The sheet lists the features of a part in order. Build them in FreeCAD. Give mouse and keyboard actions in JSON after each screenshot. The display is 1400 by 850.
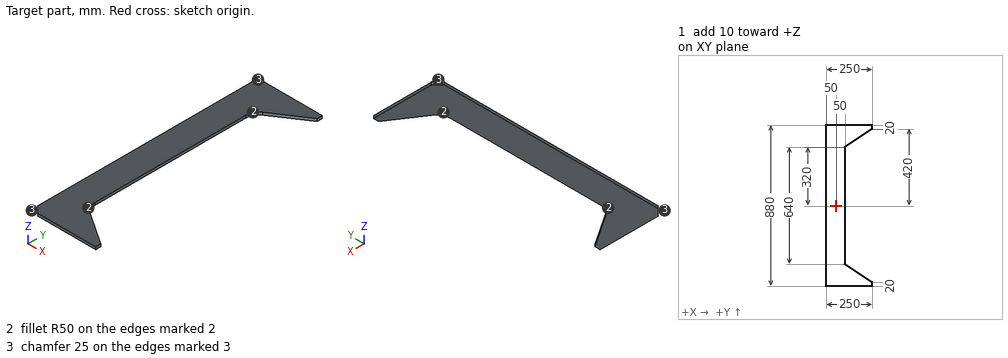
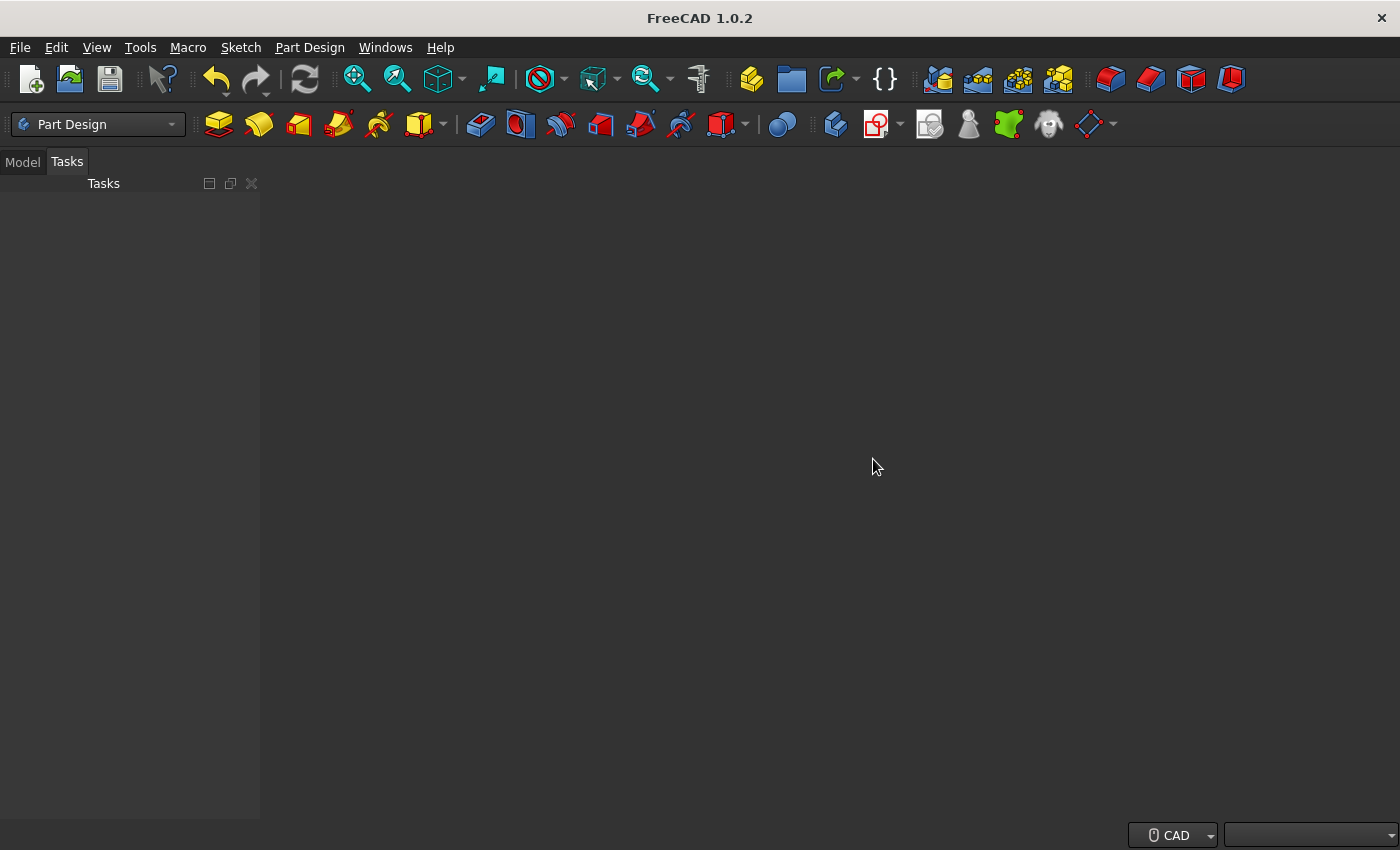
{"action": "key", "text": "ctrl+n"}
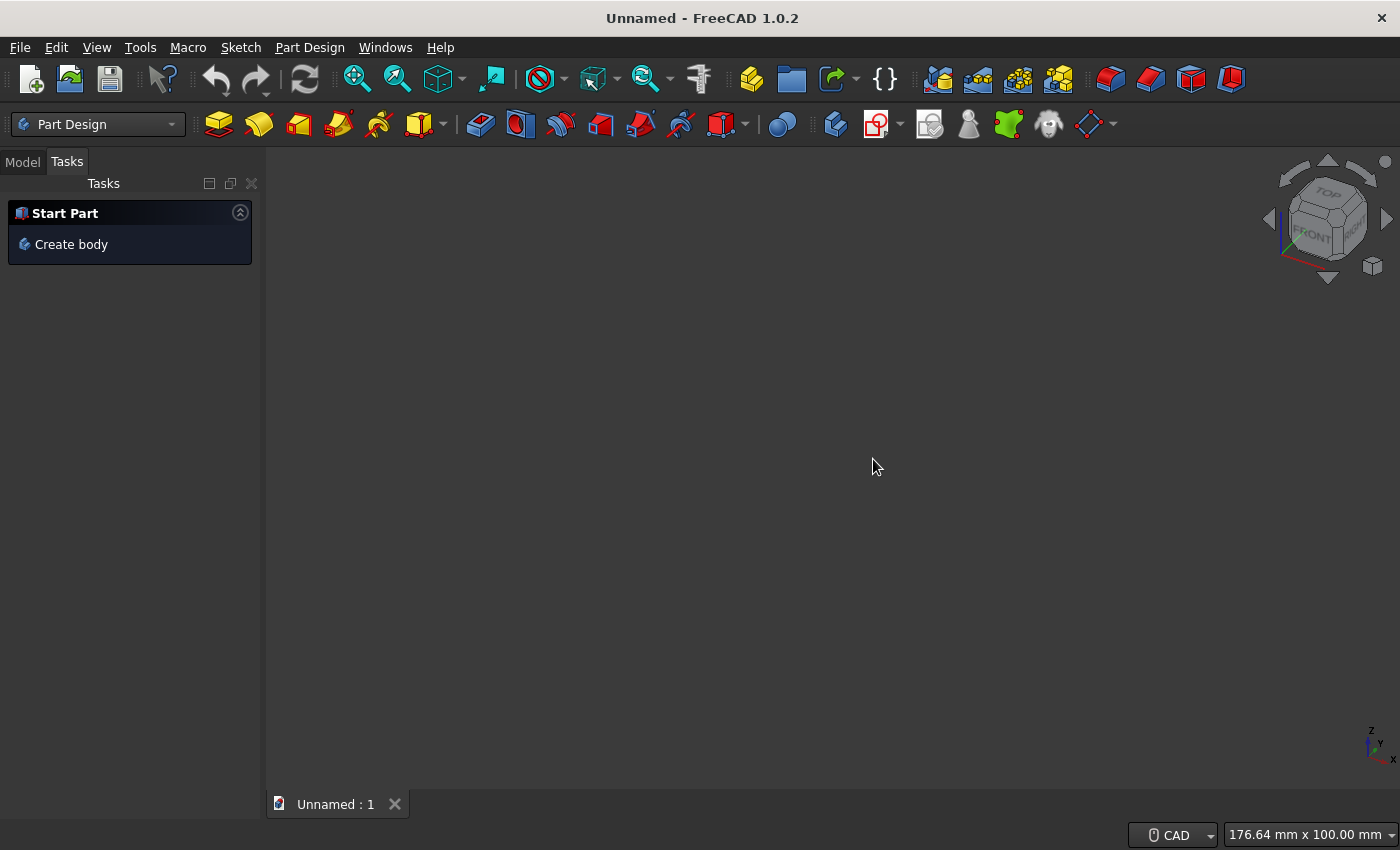
{"action": "left_click", "coordinate": [876, 124]}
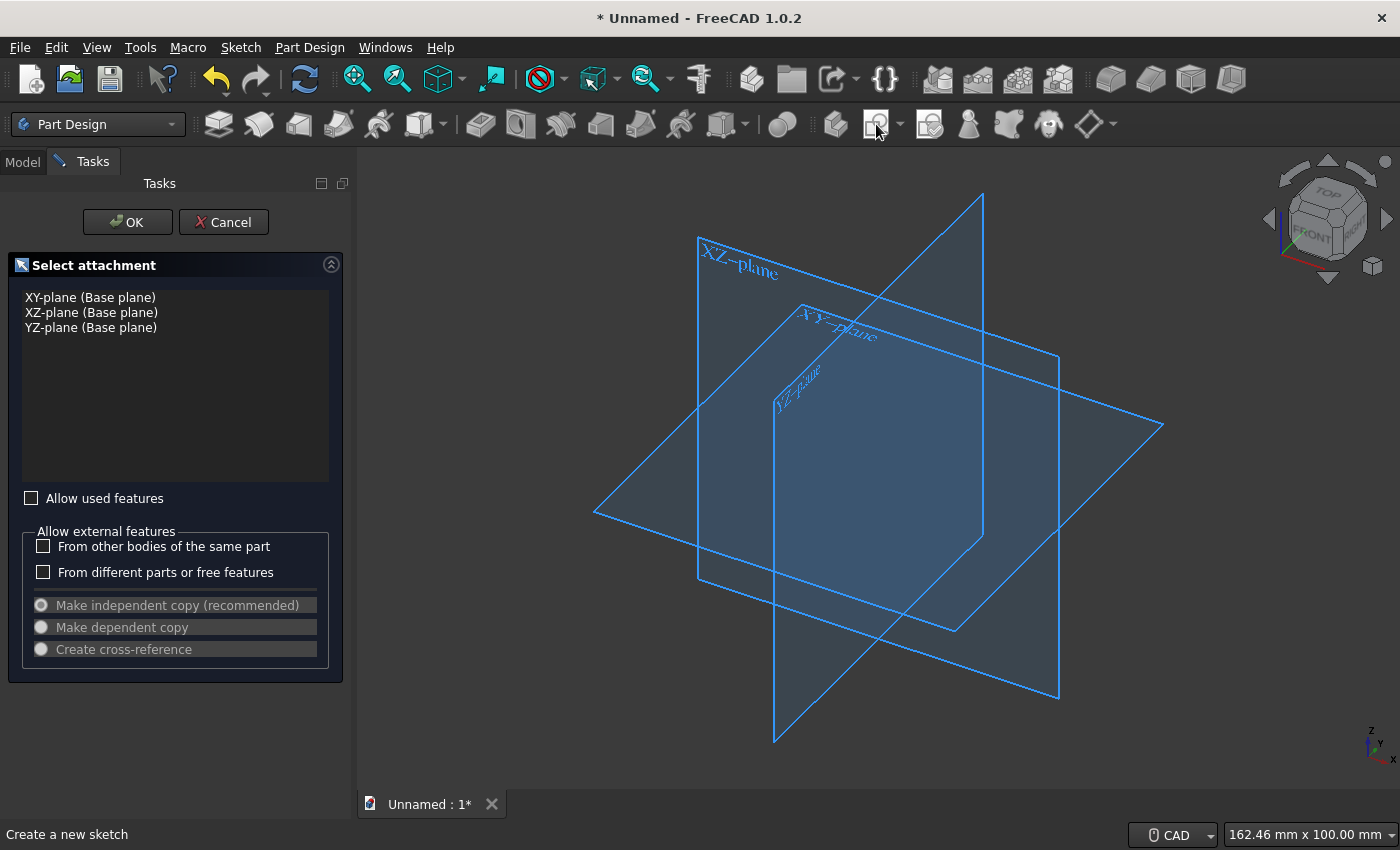
{"action": "left_click", "coordinate": [82, 298]}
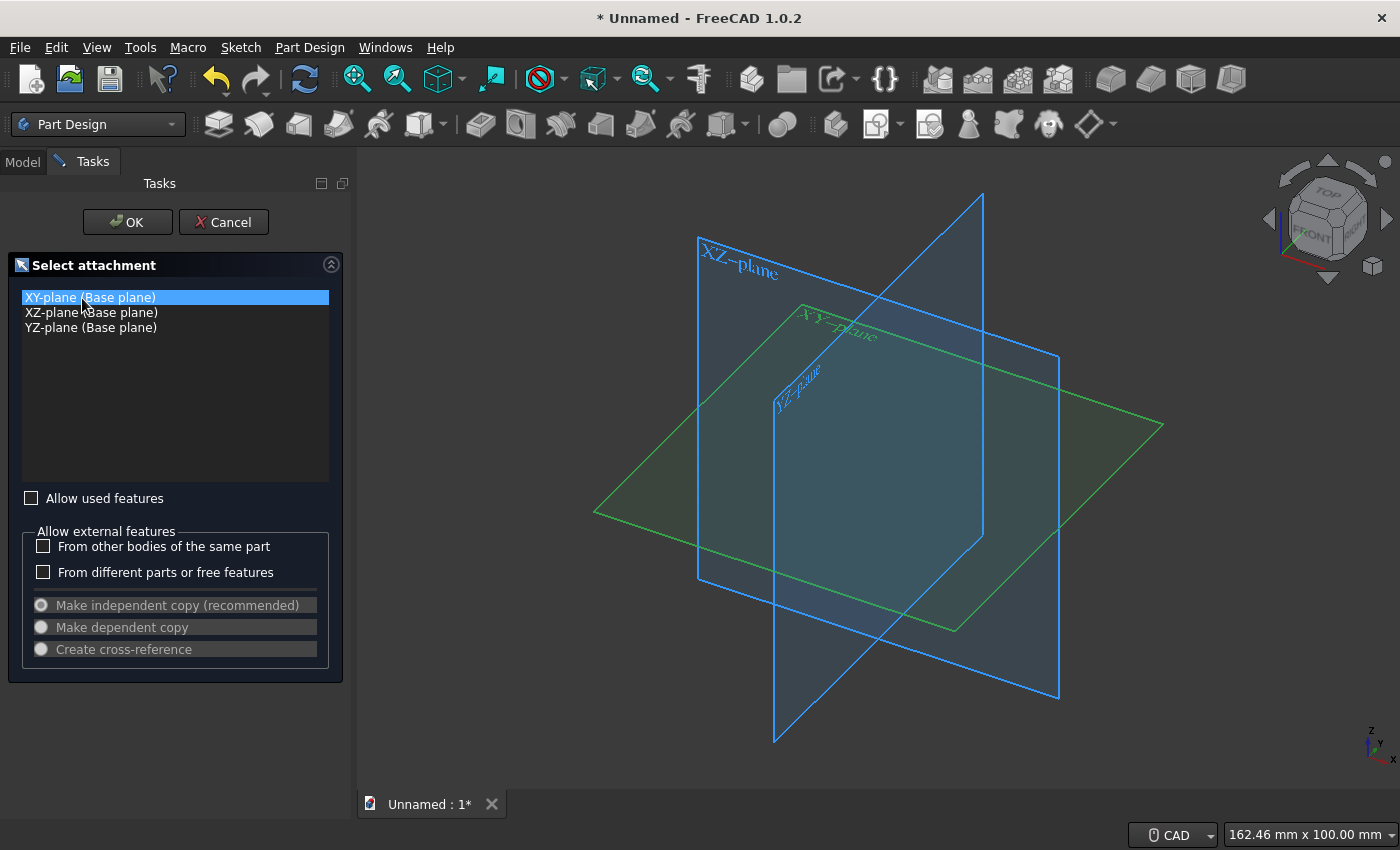
{"action": "left_click", "coordinate": [128, 222]}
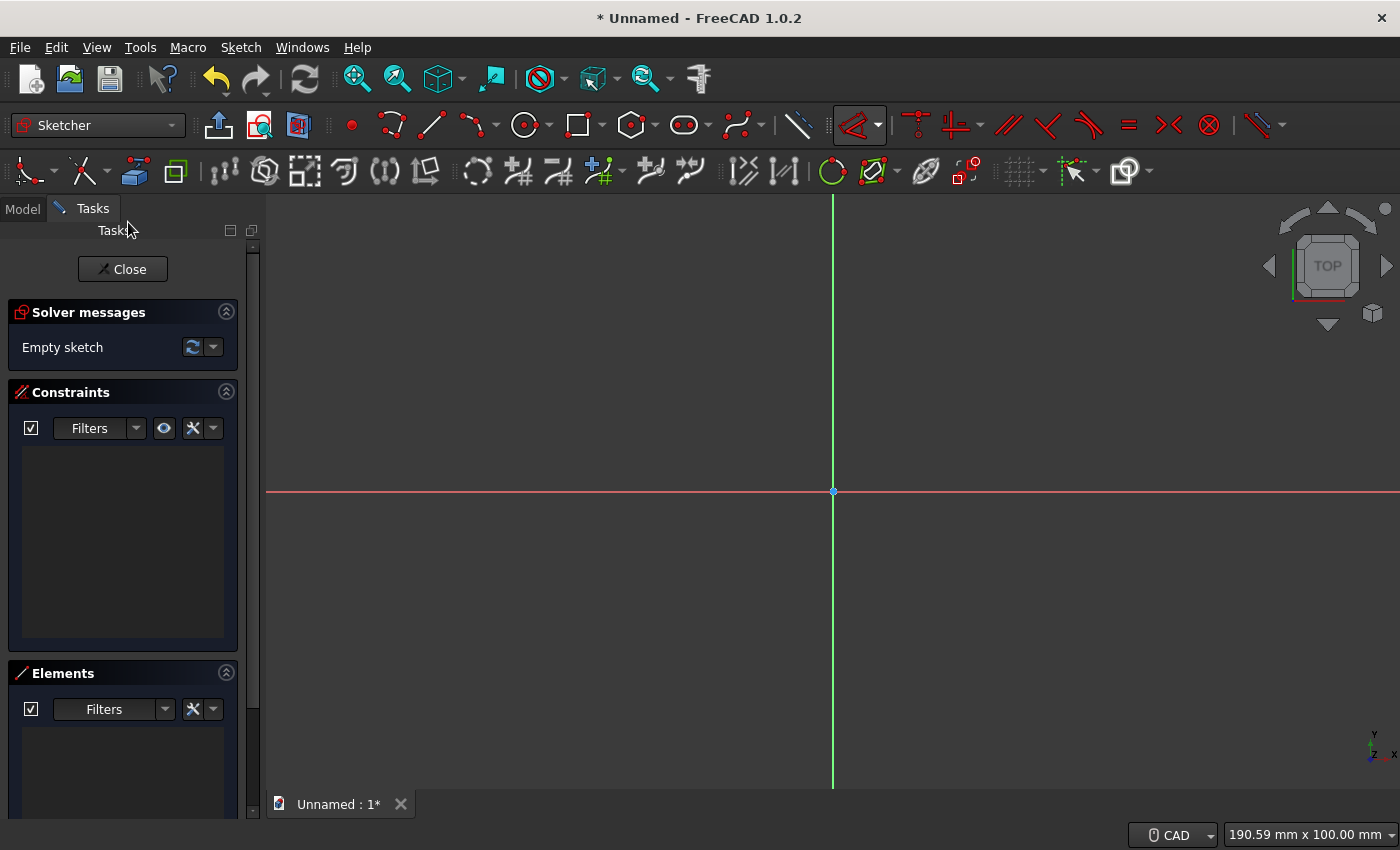
{"action": "scroll", "coordinate": [723, 492], "scroll_direction": "down", "scroll_amount": 13}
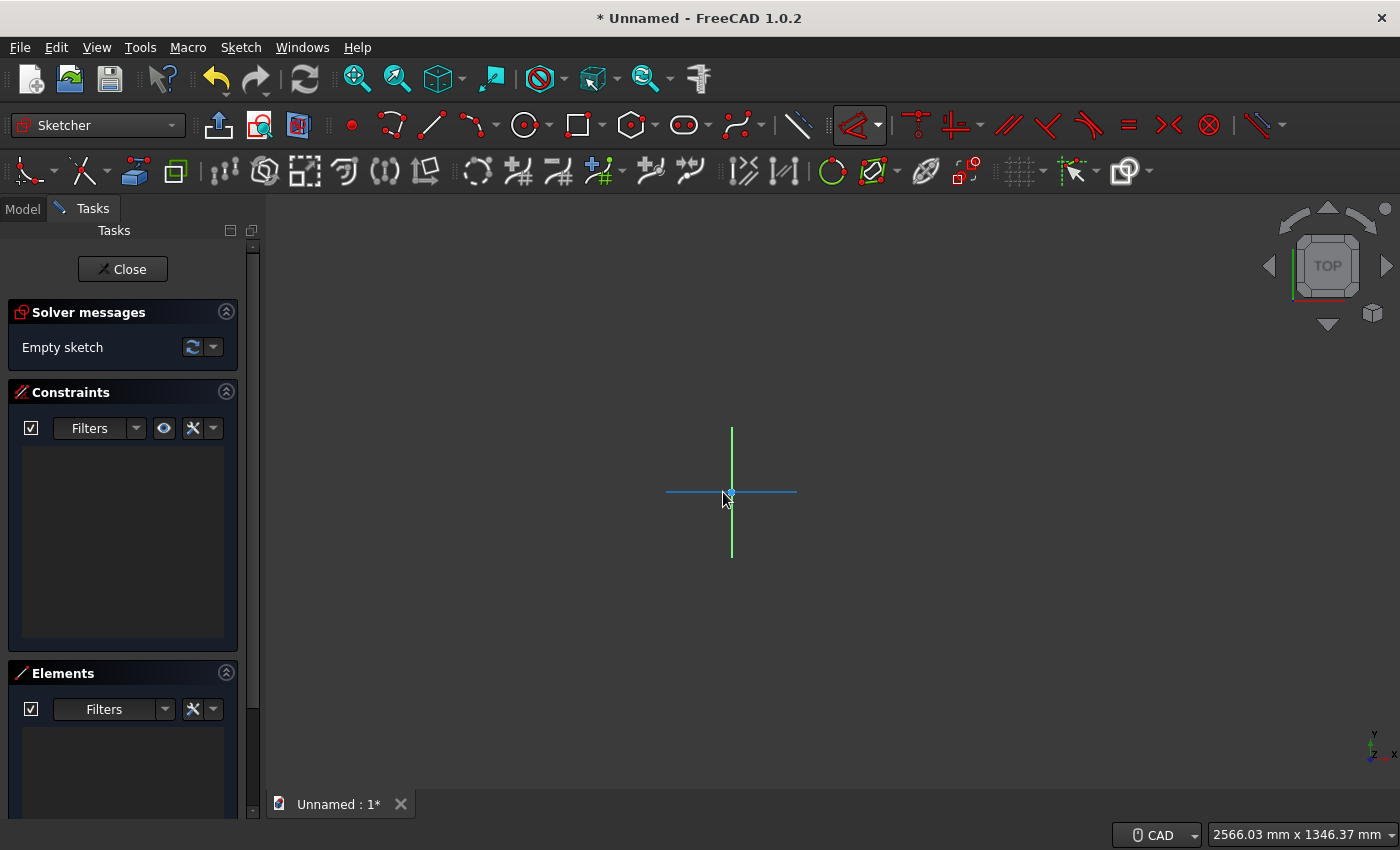
{"action": "key", "text": "g m"}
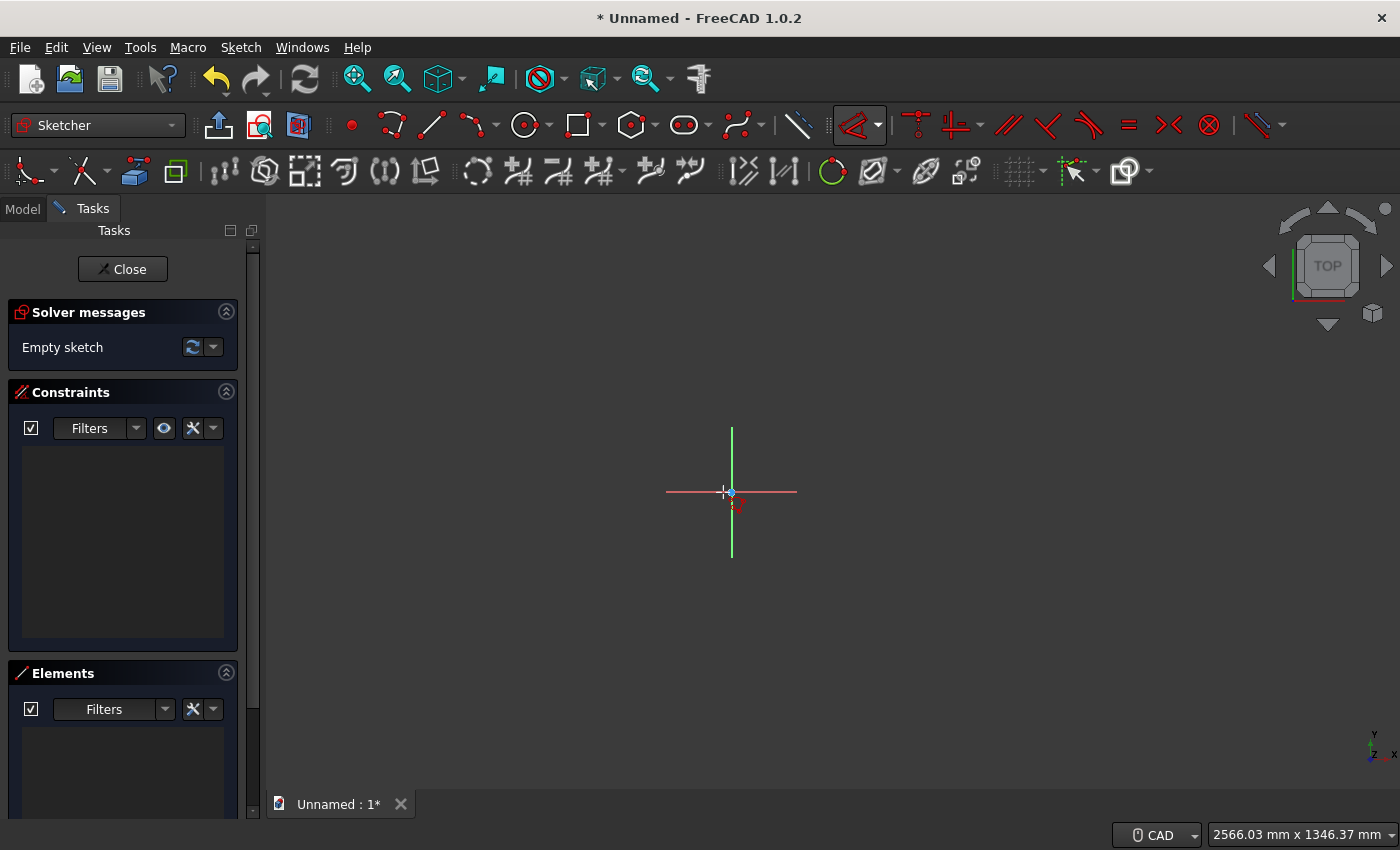
{"action": "left_click", "coordinate": [754, 351]}
{"action": "left_click", "coordinate": [820, 307]}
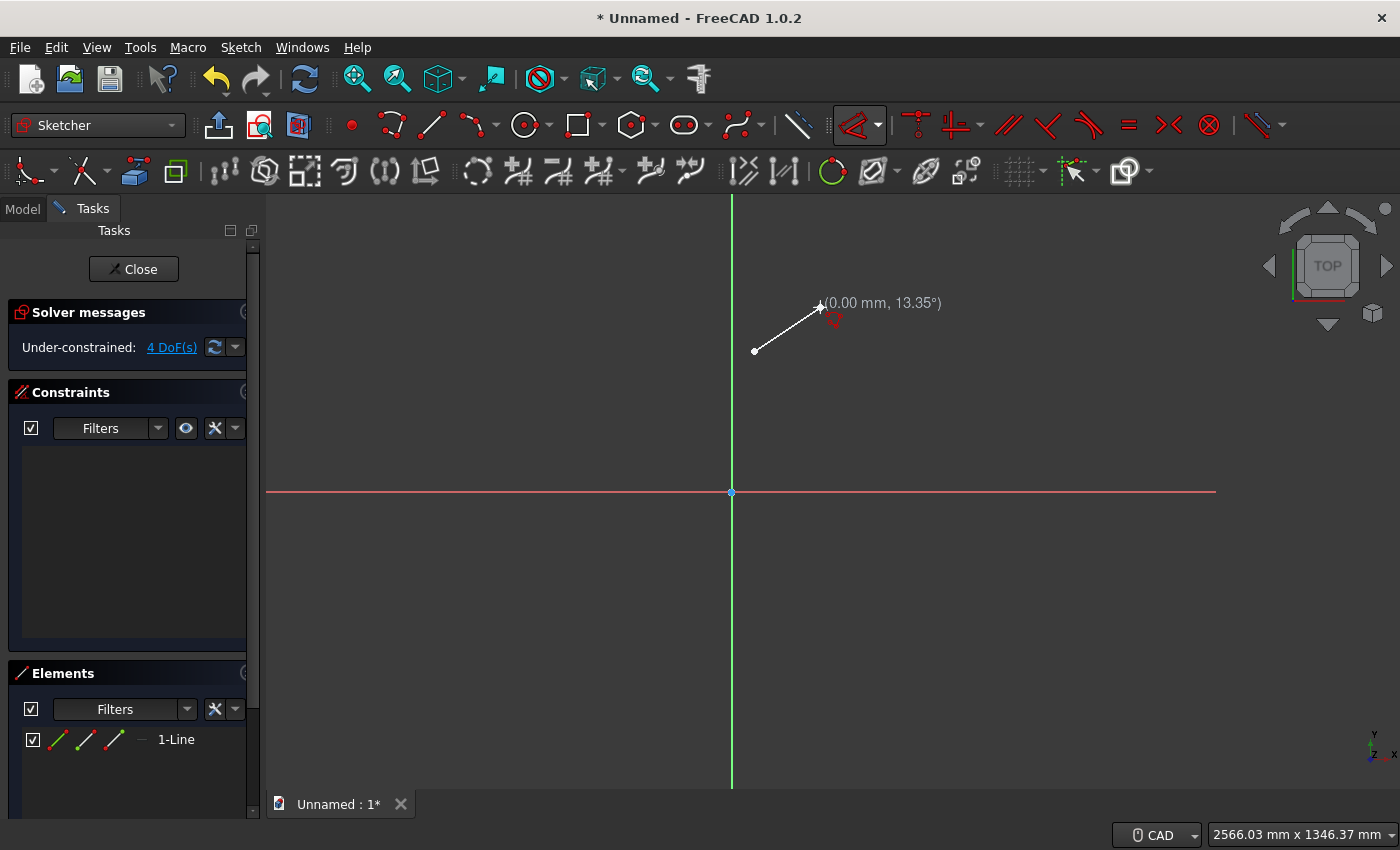
{"action": "scroll", "coordinate": [820, 298], "scroll_direction": "up", "scroll_amount": 3}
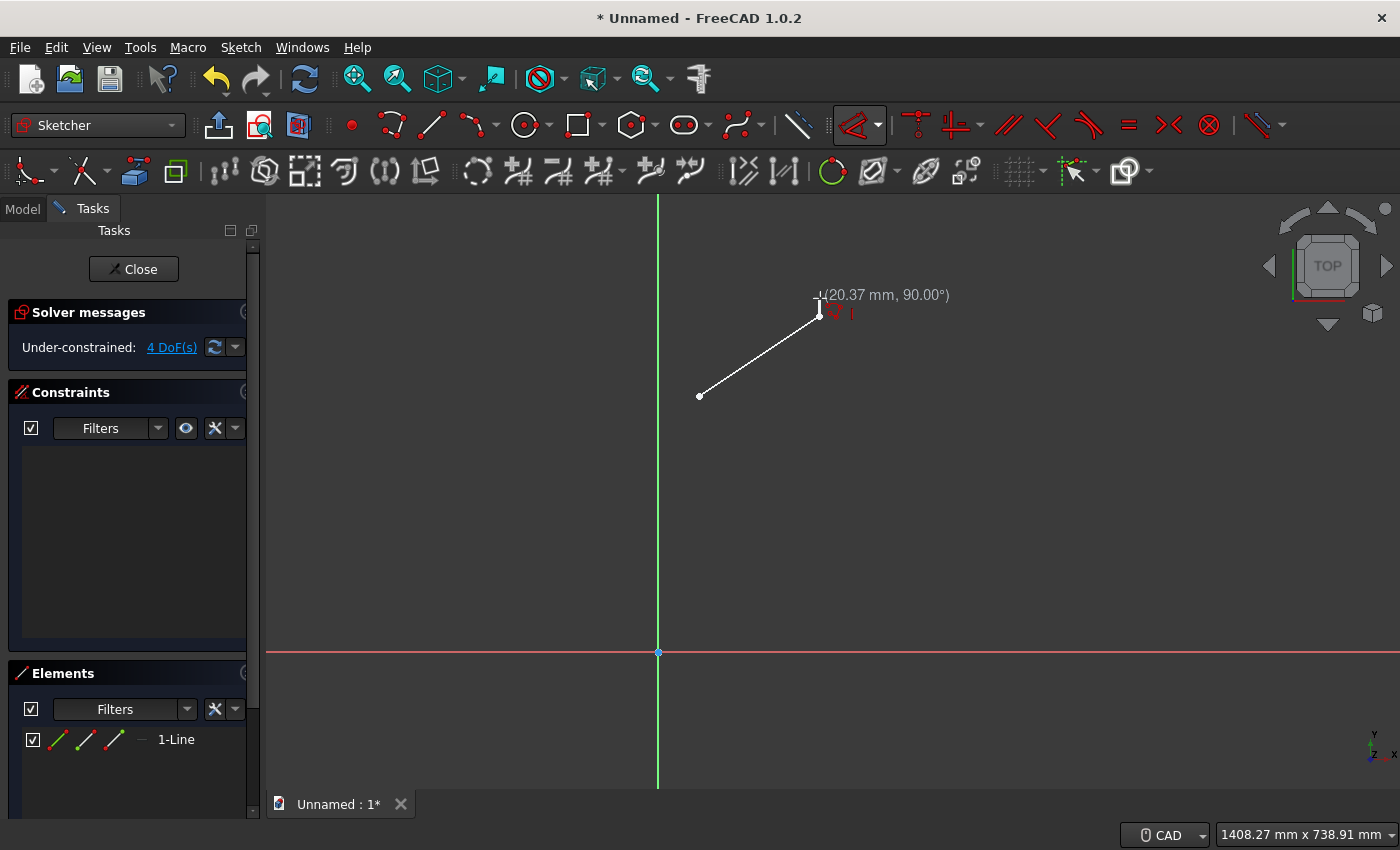
{"action": "left_click", "coordinate": [820, 298]}
{"action": "left_click", "coordinate": [618, 298]}